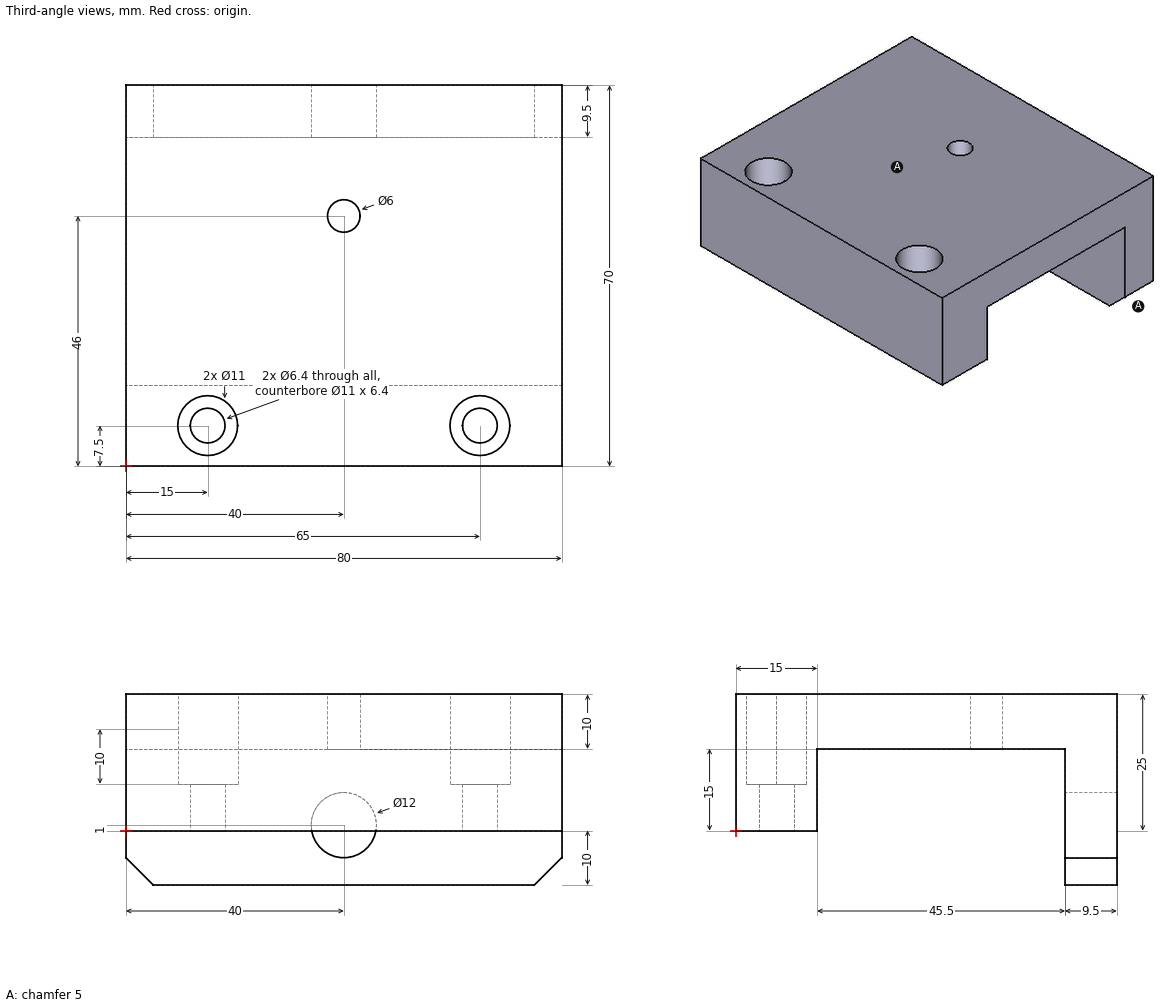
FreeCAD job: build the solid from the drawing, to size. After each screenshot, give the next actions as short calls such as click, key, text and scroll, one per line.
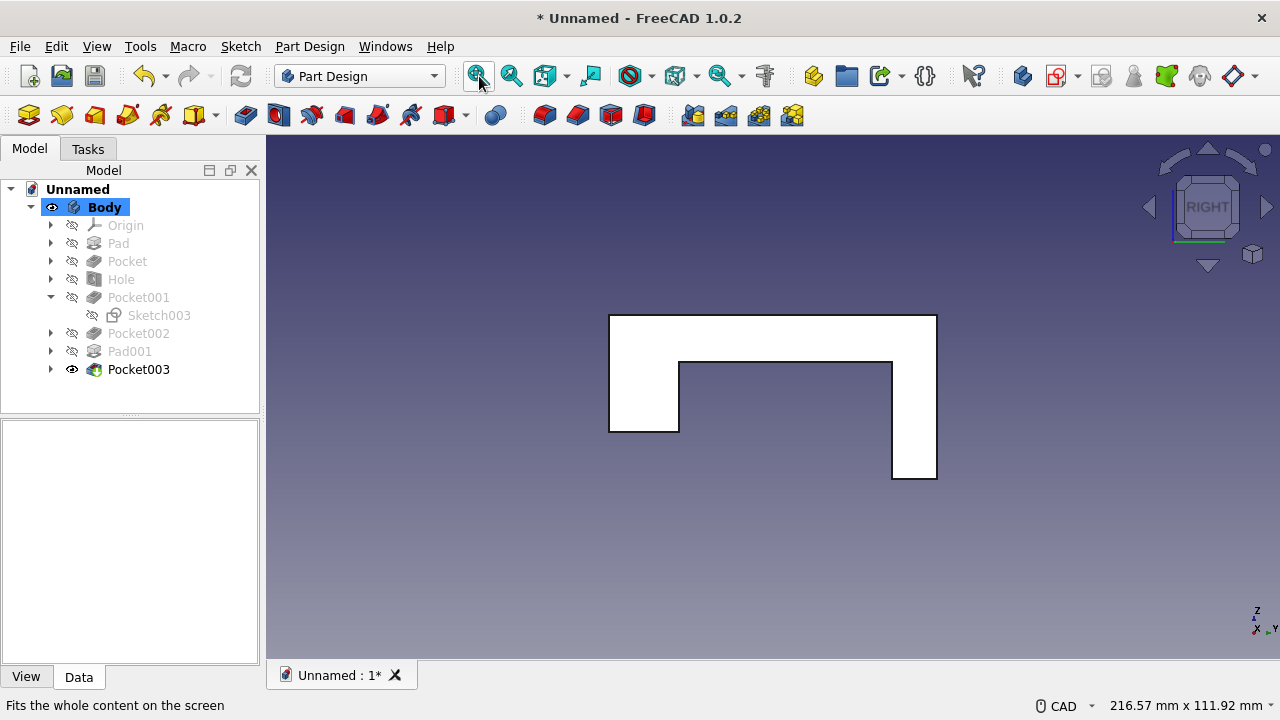
click(915, 478)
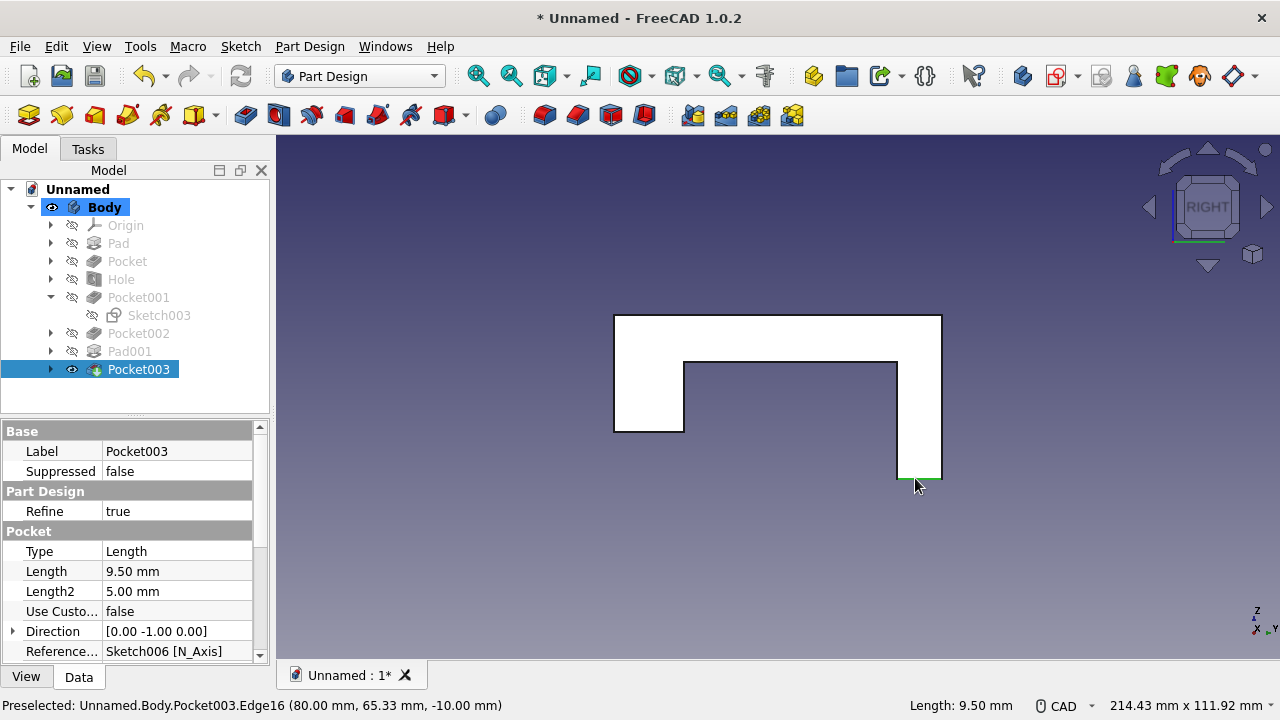
key(5)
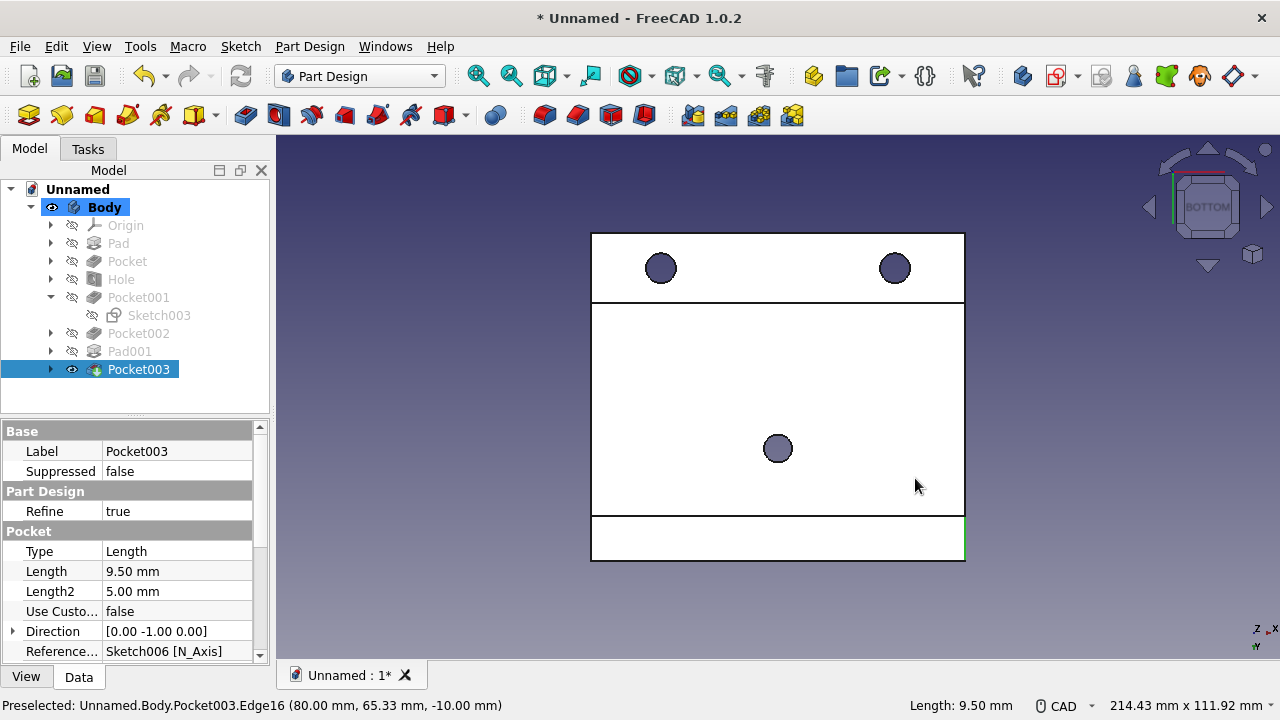
click(591, 538, ctrl)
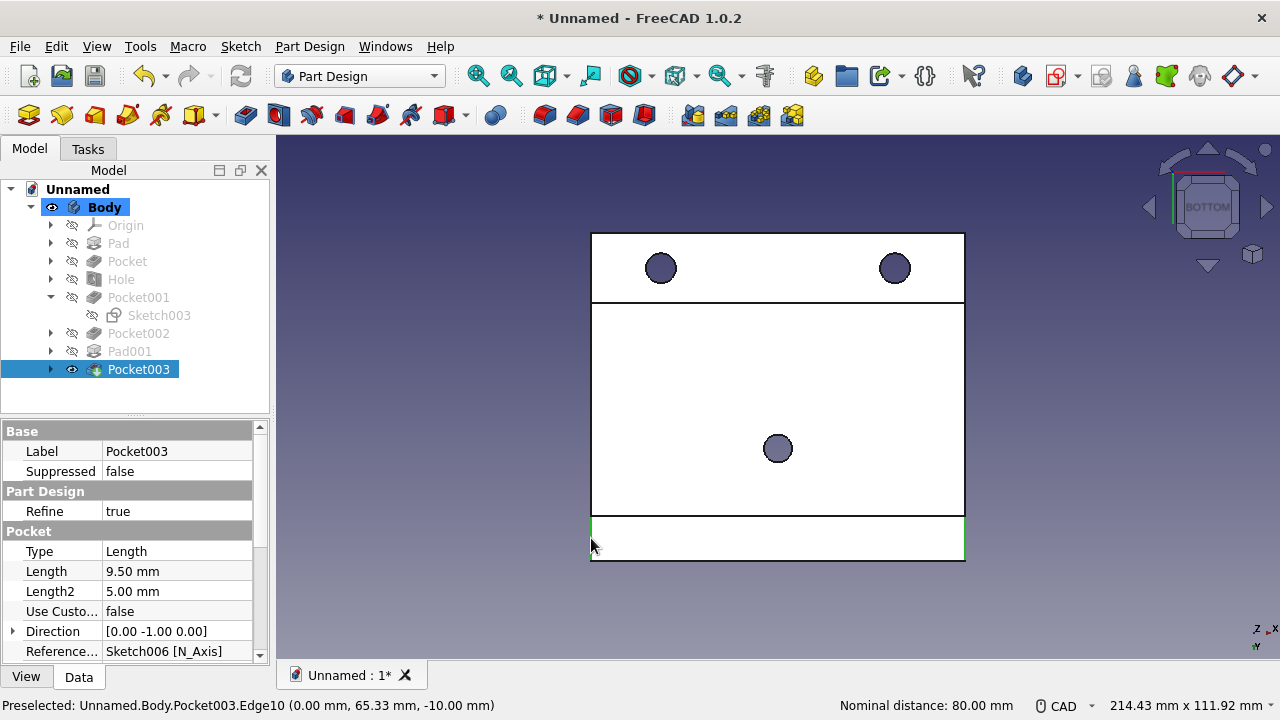
click(578, 116)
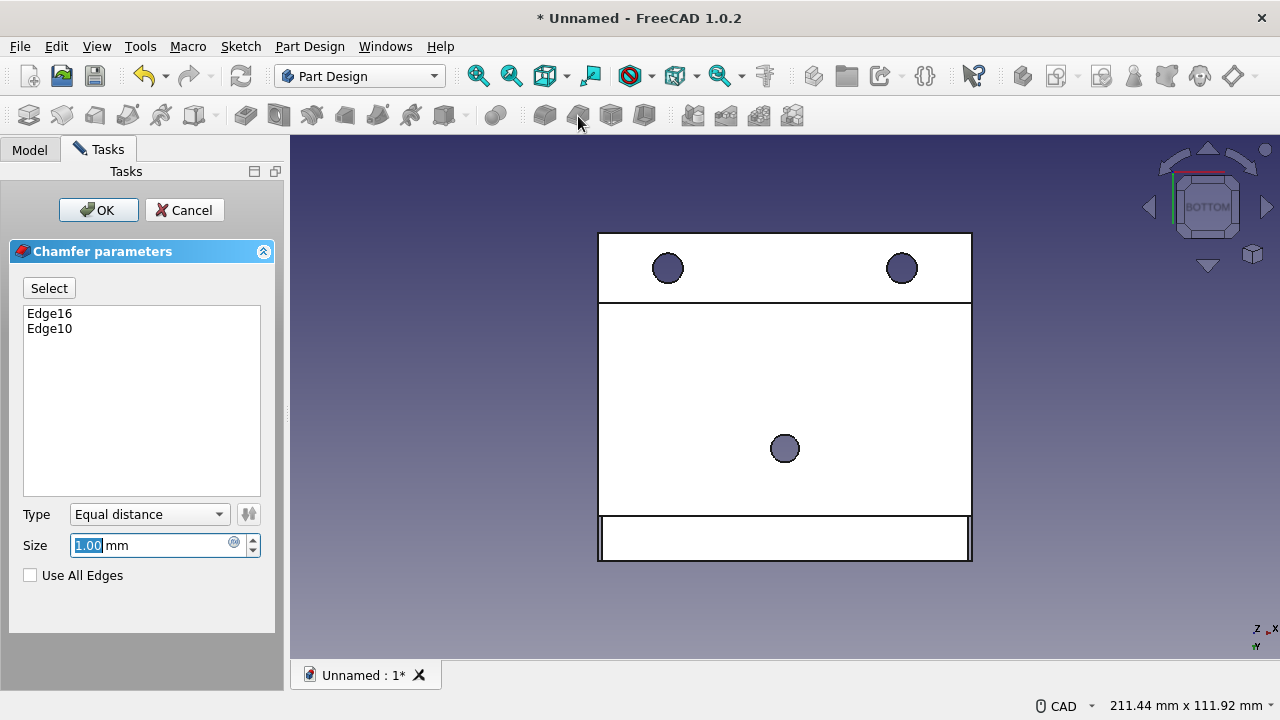
text(5)
key(Tab)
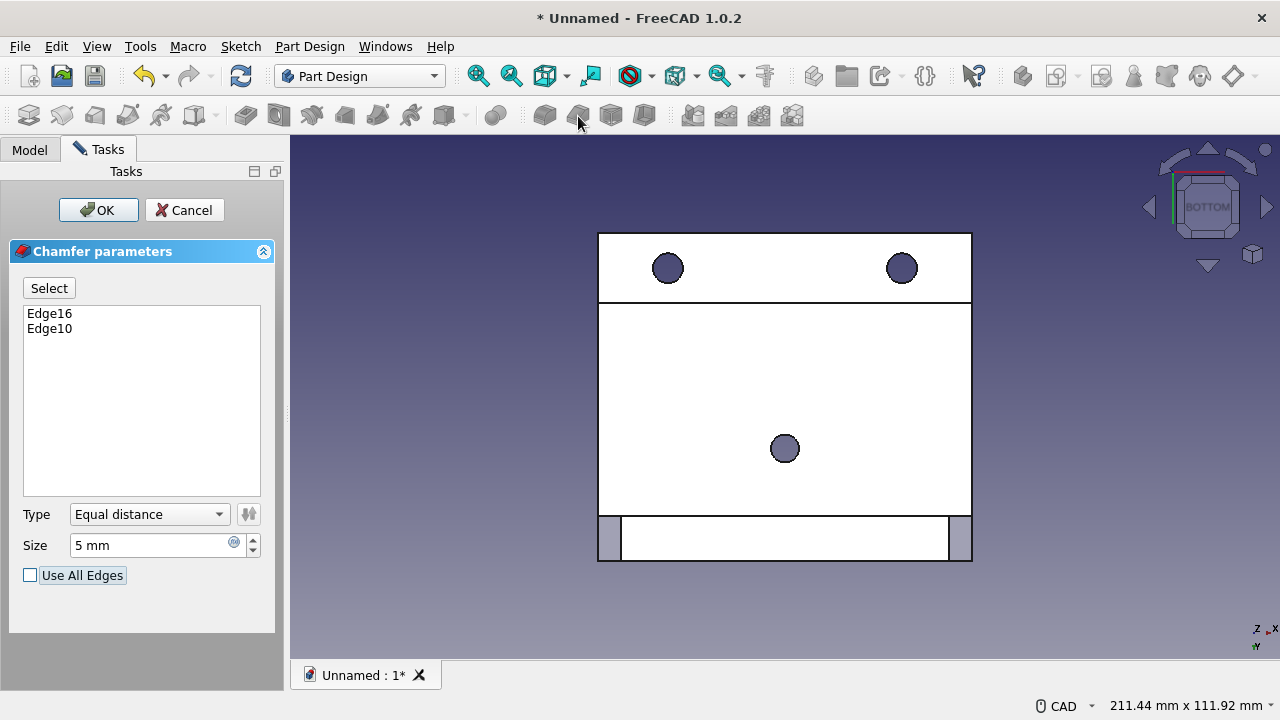
click(99, 210)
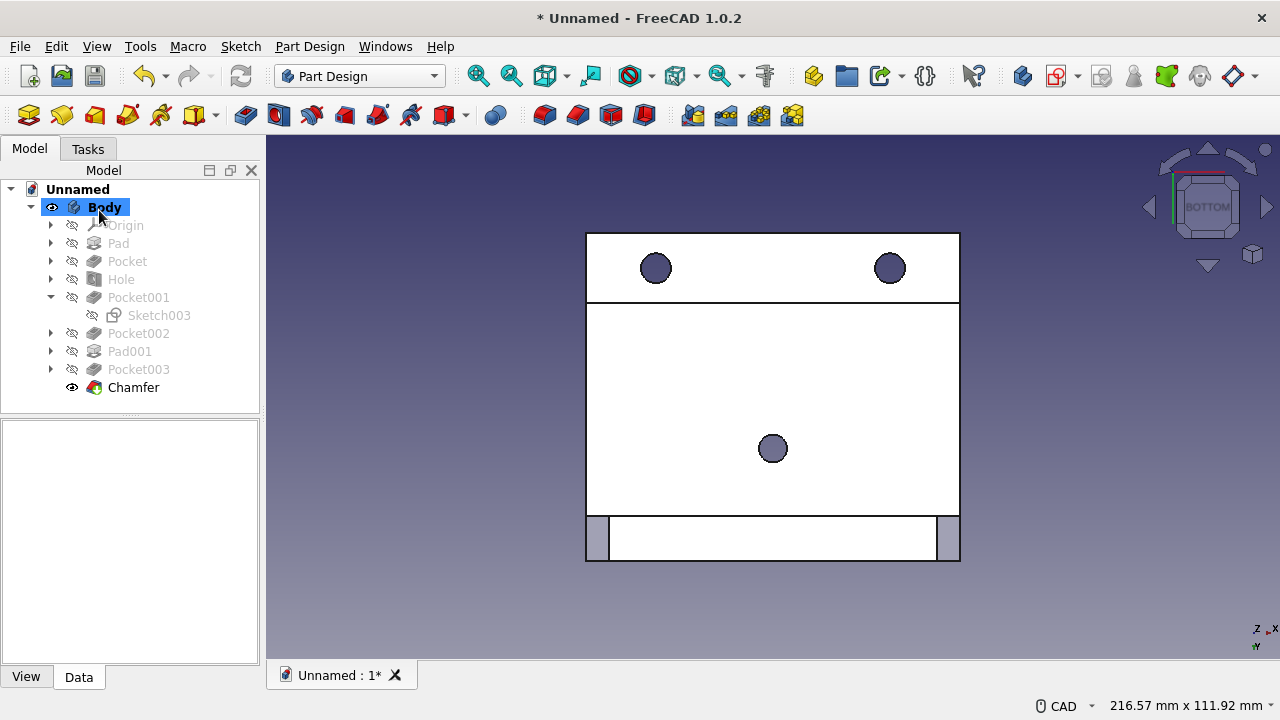
key(0)